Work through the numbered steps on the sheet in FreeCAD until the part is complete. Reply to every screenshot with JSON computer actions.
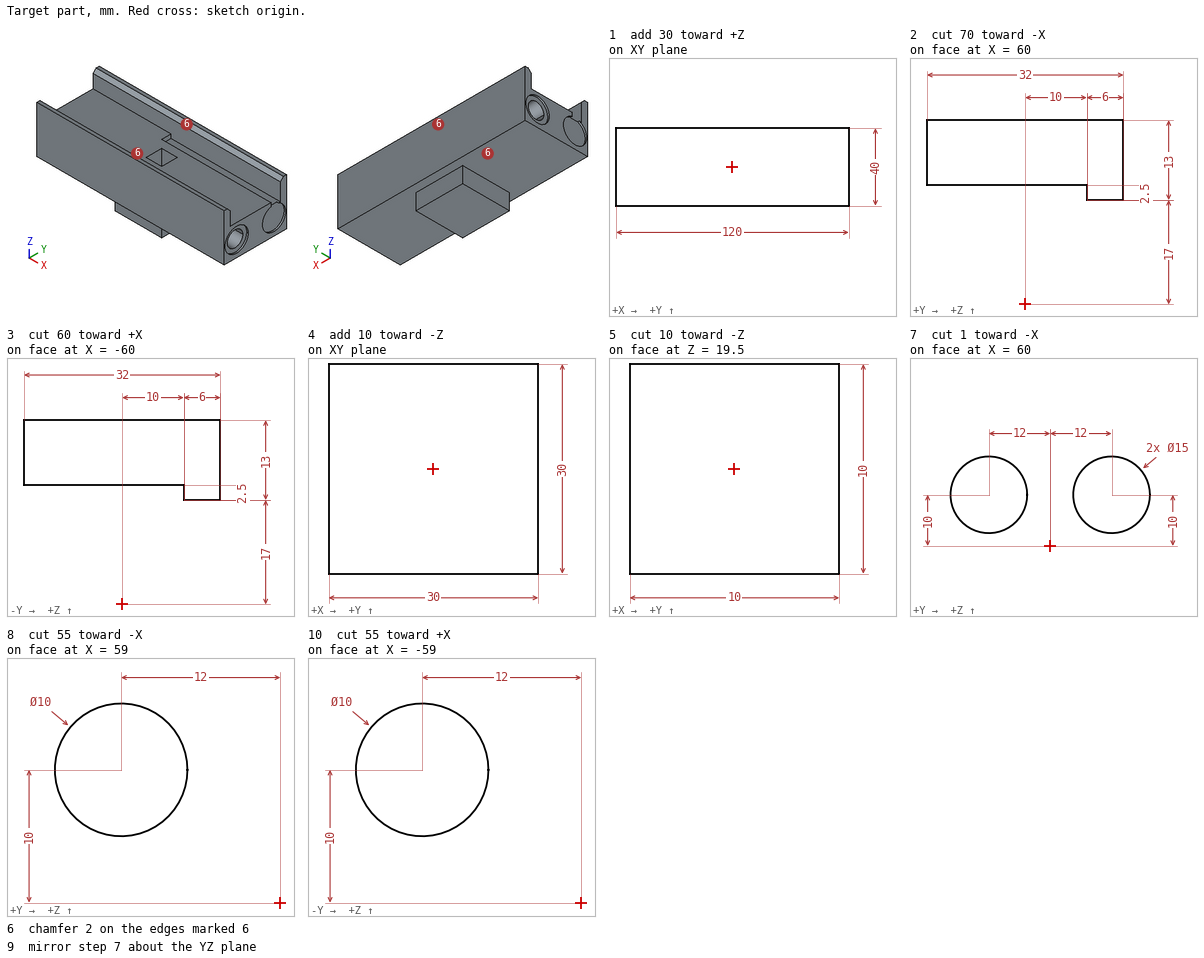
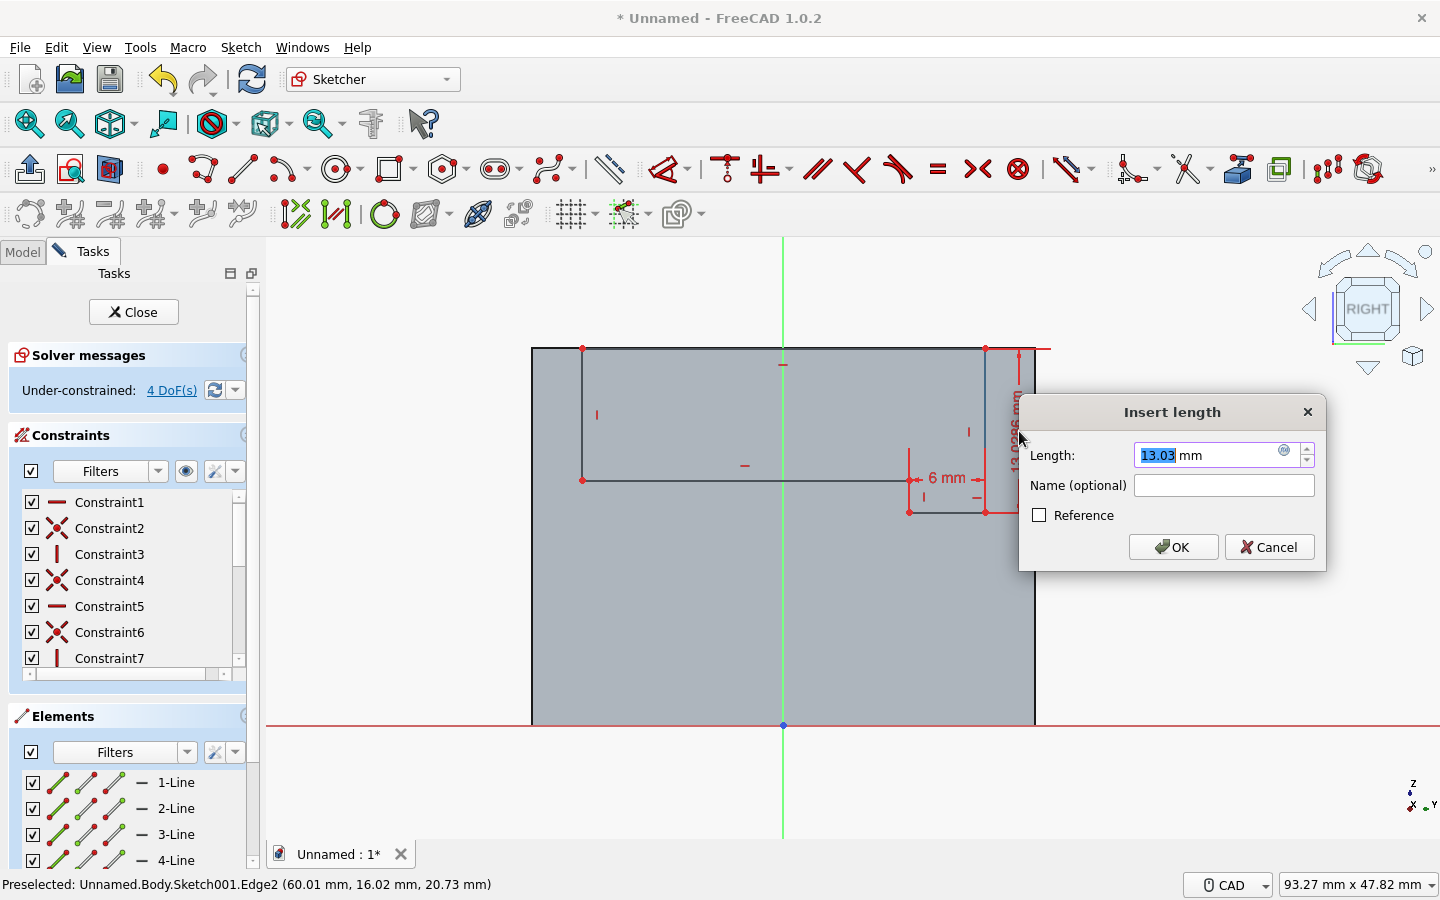
{"action": "type", "text": "13"}
{"action": "key", "text": "Return"}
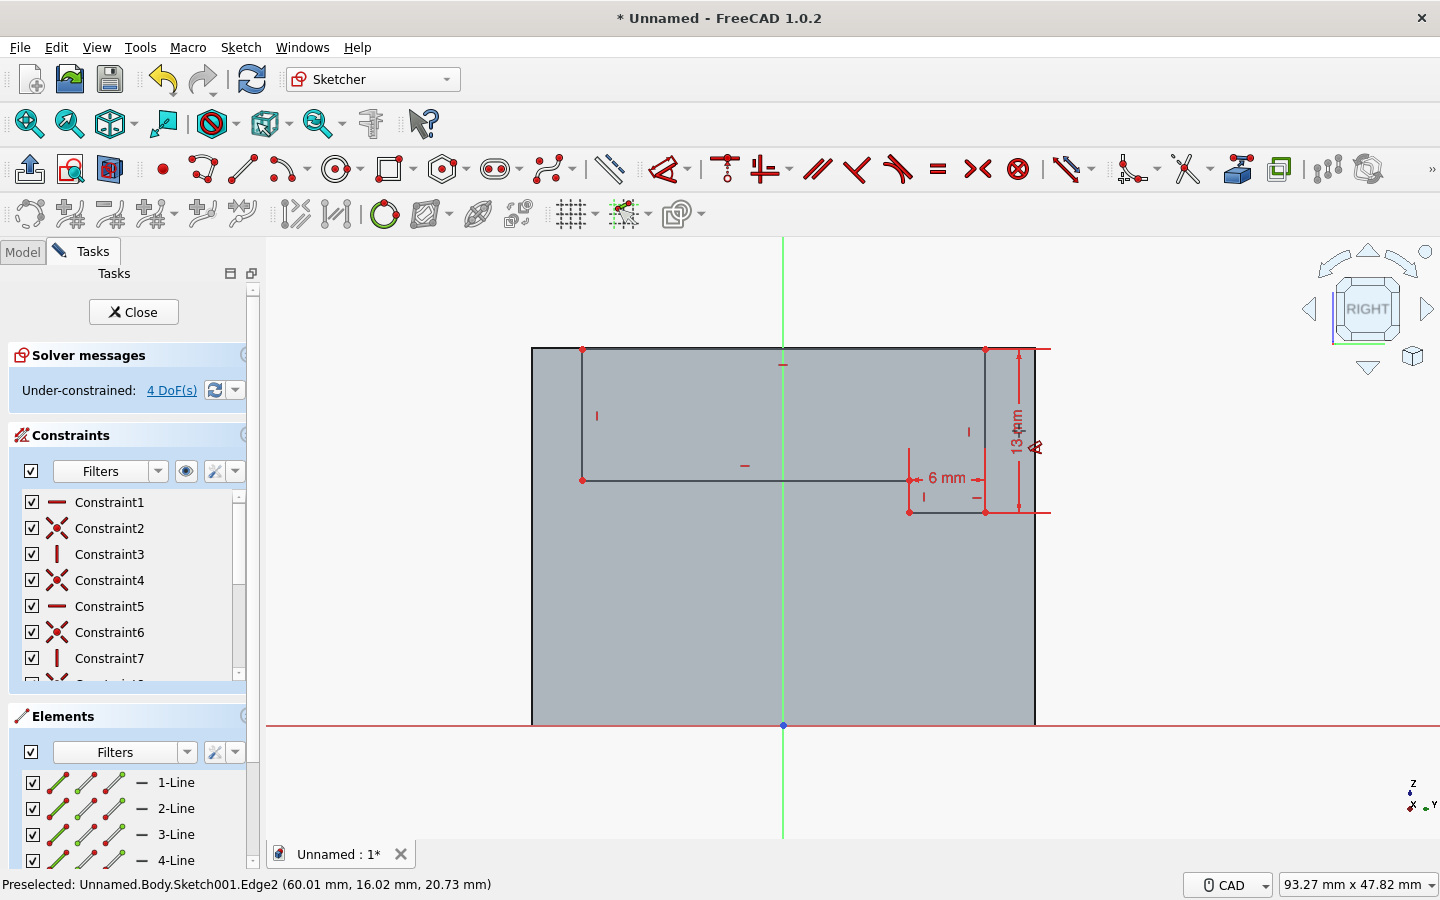
{"action": "left_click", "coordinate": [864, 349]}
{"action": "left_click", "coordinate": [691, 315]}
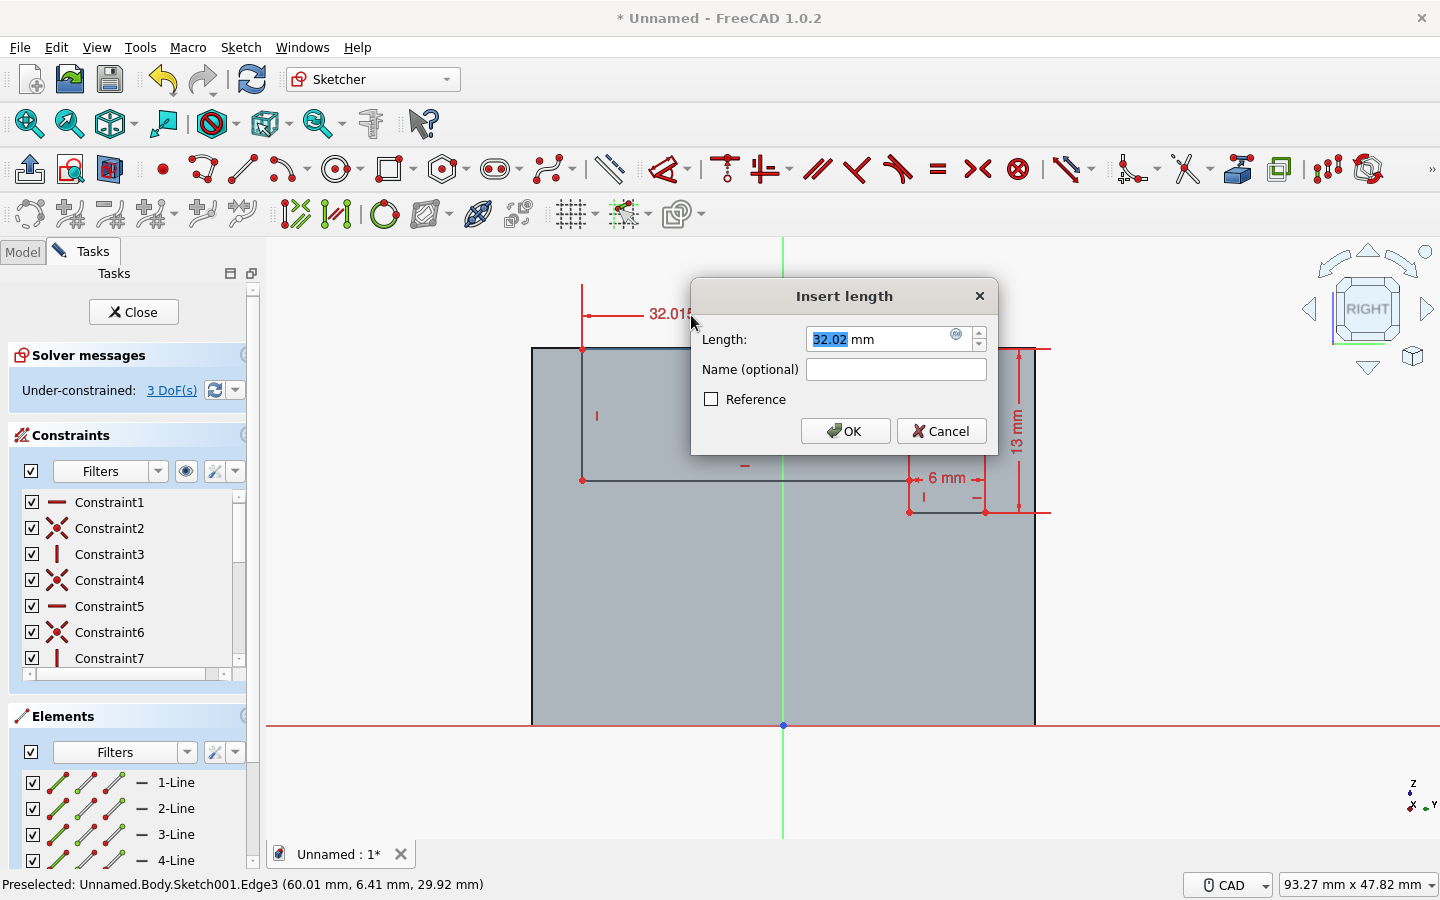
{"action": "type", "text": "32"}
{"action": "key", "text": "Return"}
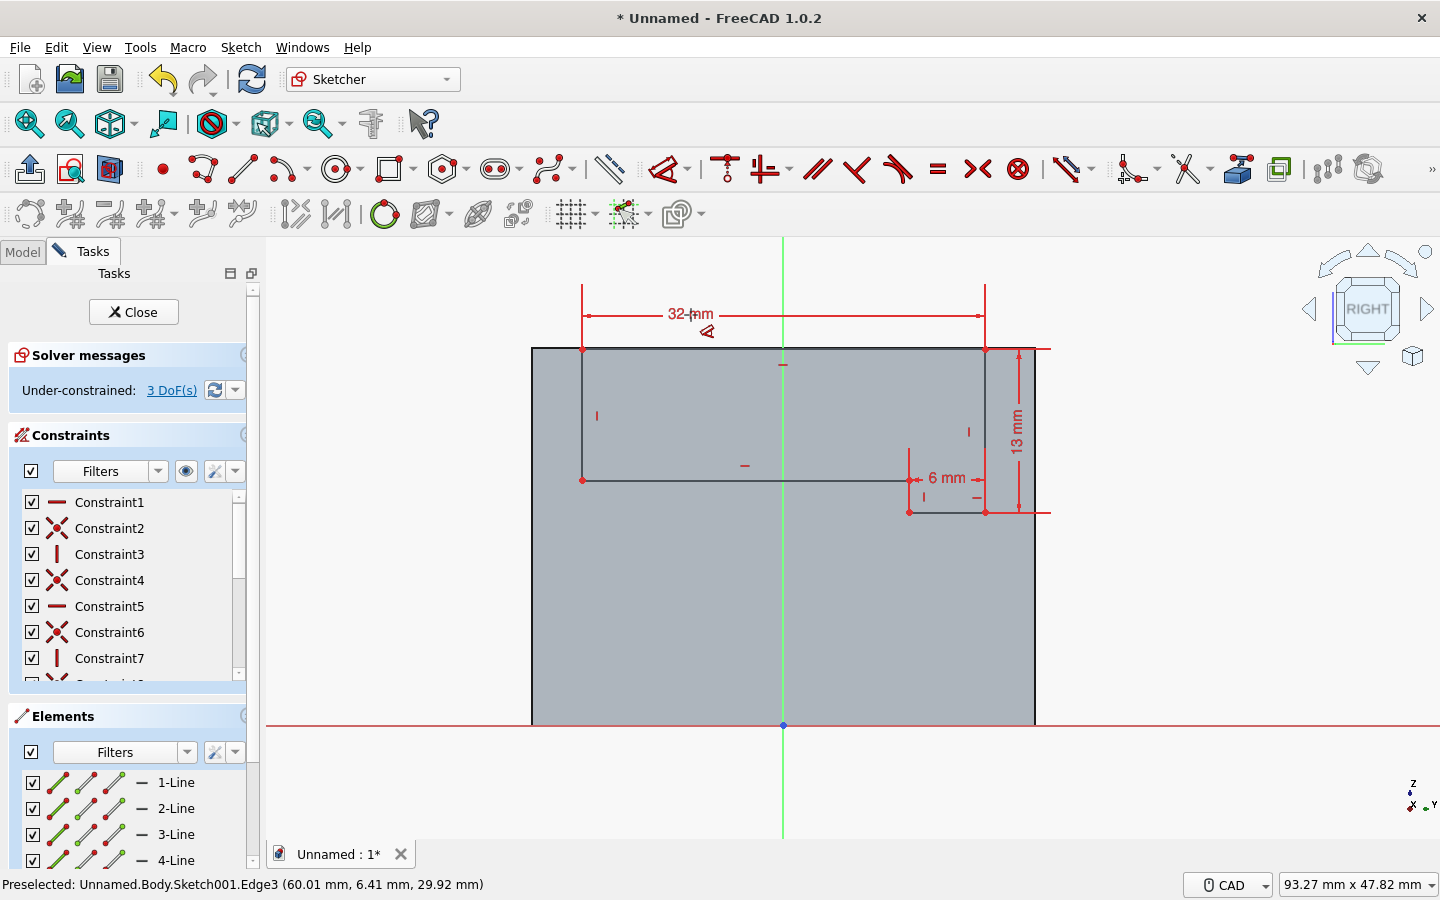
{"action": "scroll", "coordinate": [909, 491], "scroll_direction": "up", "scroll_amount": 2}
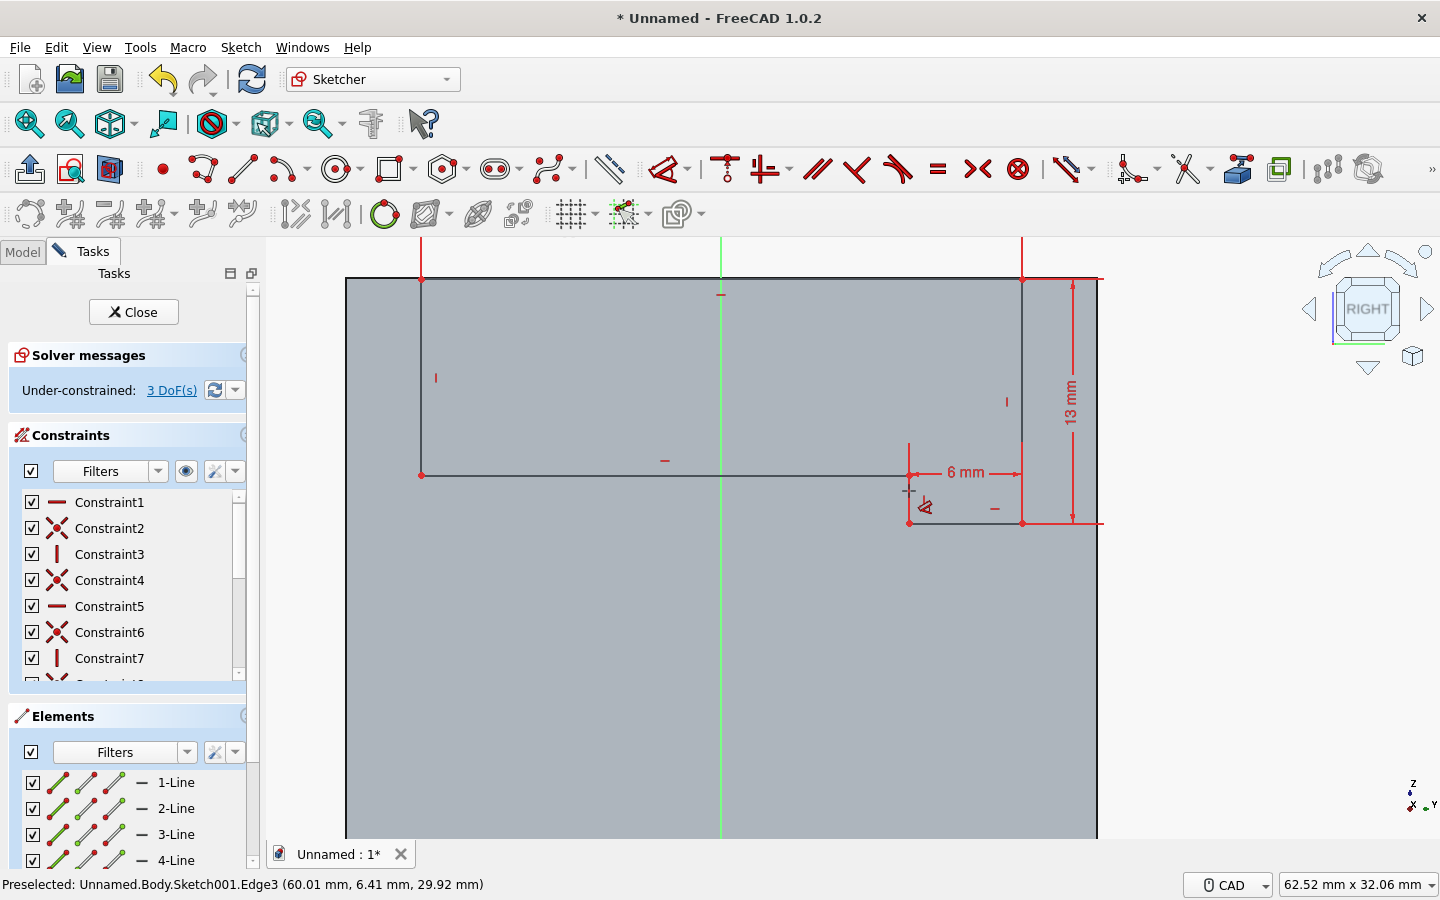
{"action": "left_click", "coordinate": [909, 490]}
{"action": "left_click", "coordinate": [943, 500]}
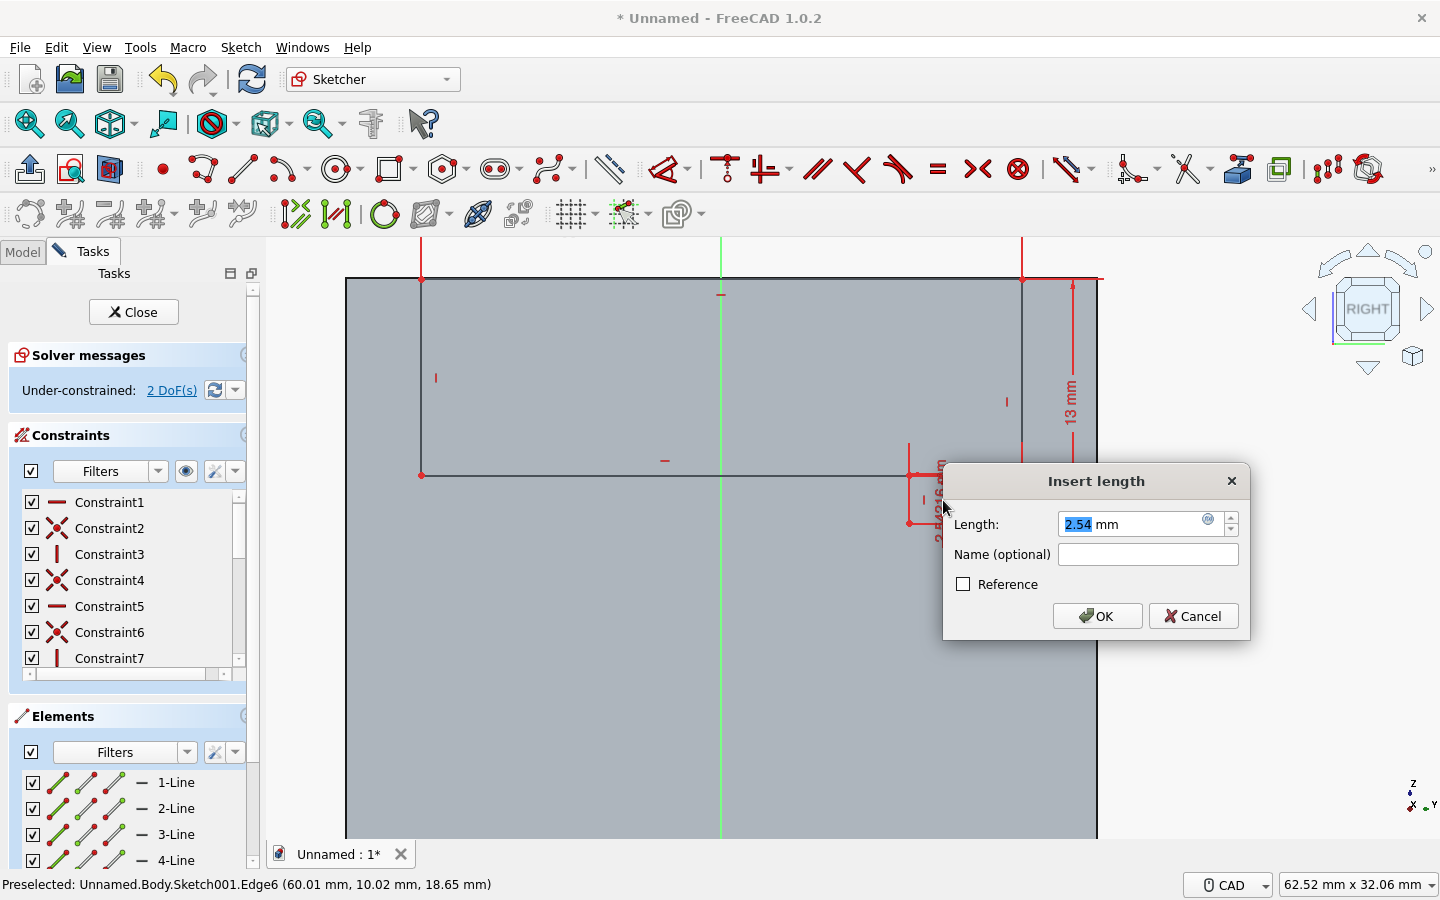
{"action": "type", "text": "2.5"}
{"action": "key", "text": "Return"}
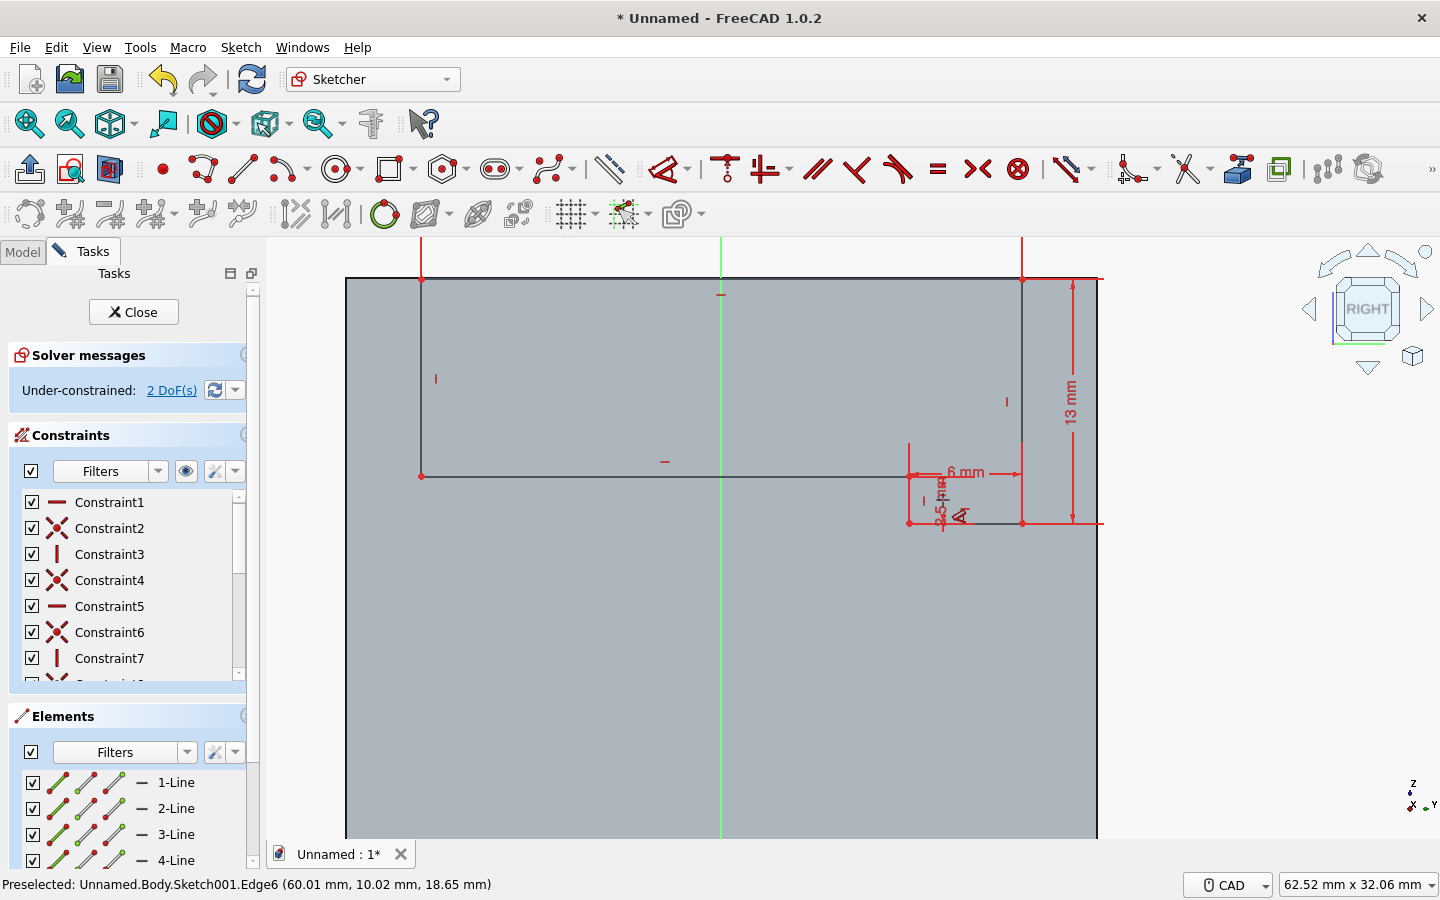
{"action": "left_click", "coordinate": [909, 524]}
{"action": "left_click", "coordinate": [815, 442]}